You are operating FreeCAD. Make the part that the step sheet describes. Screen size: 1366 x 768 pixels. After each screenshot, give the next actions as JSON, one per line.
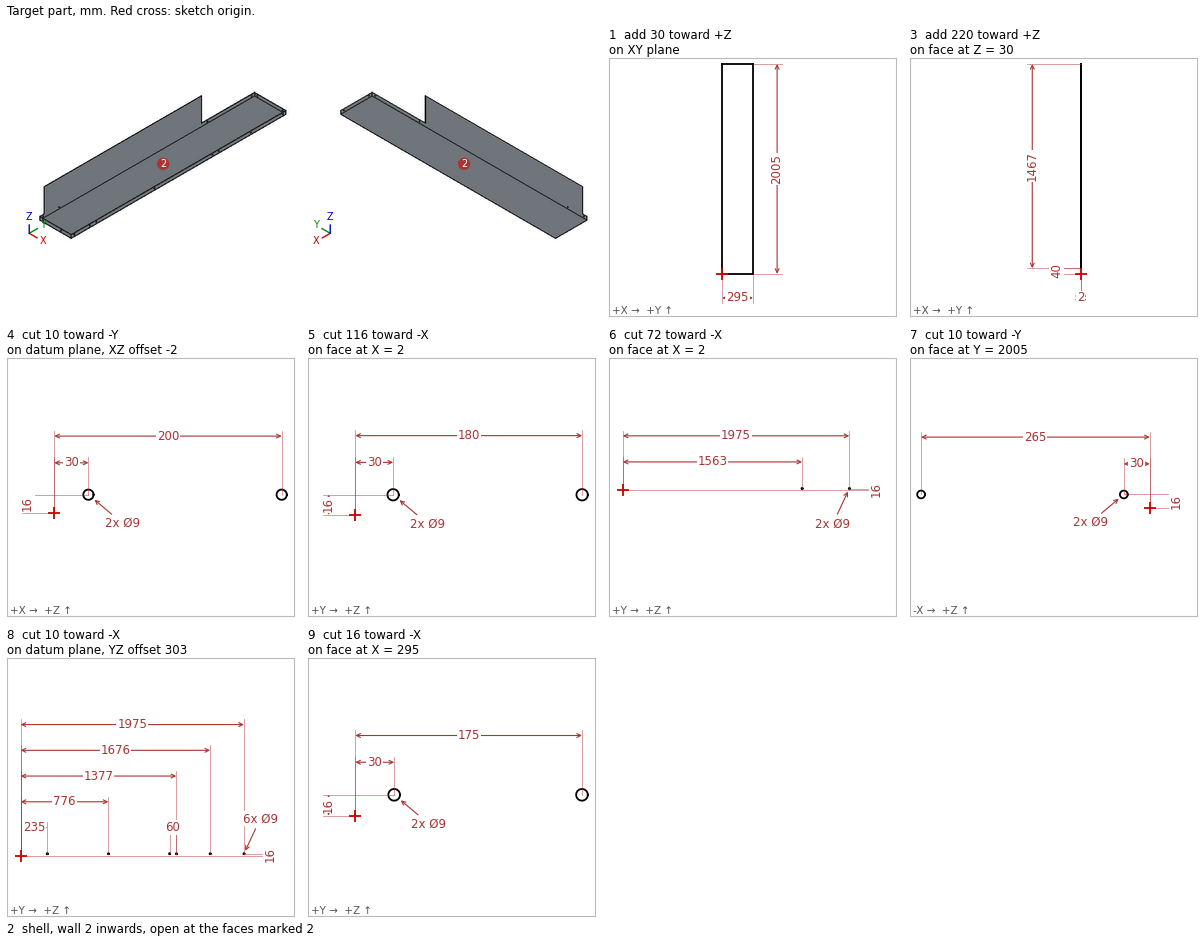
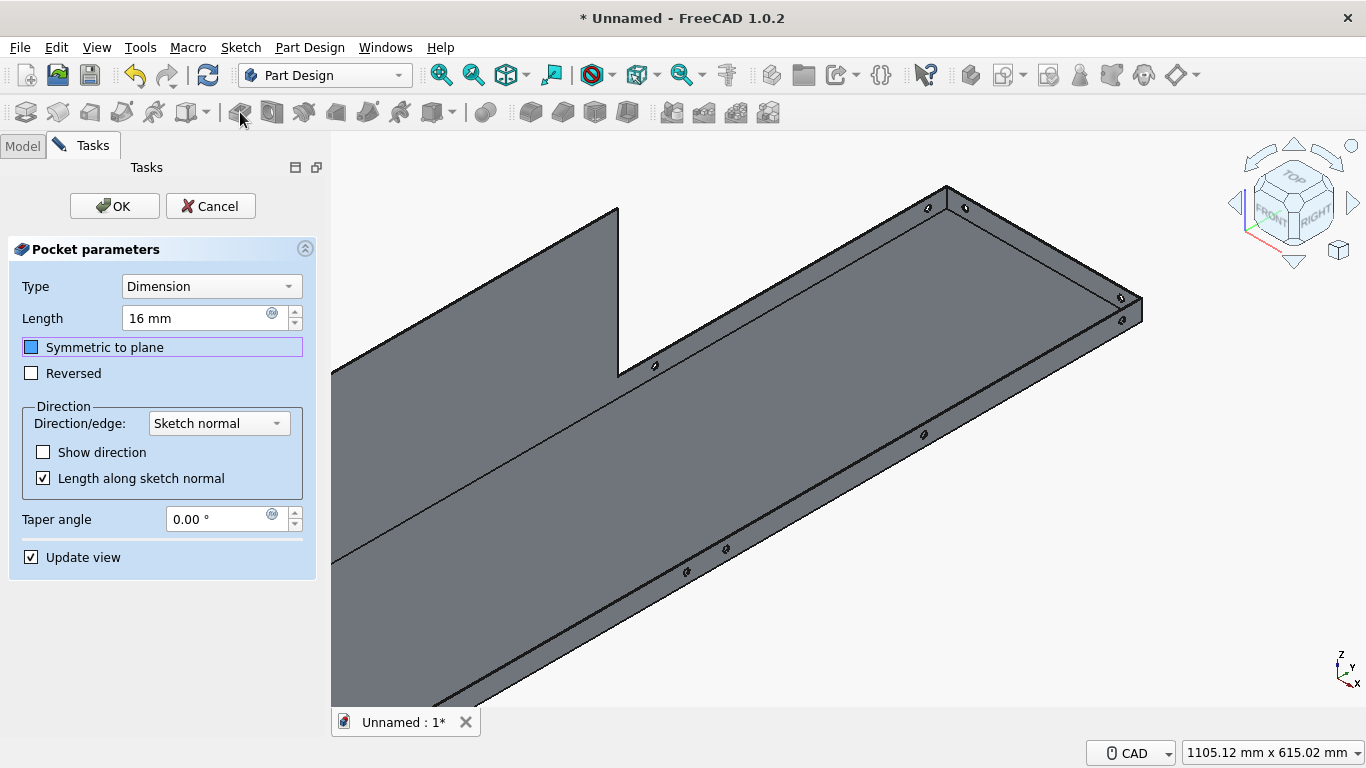
{"action": "left_click", "coordinate": [115, 206]}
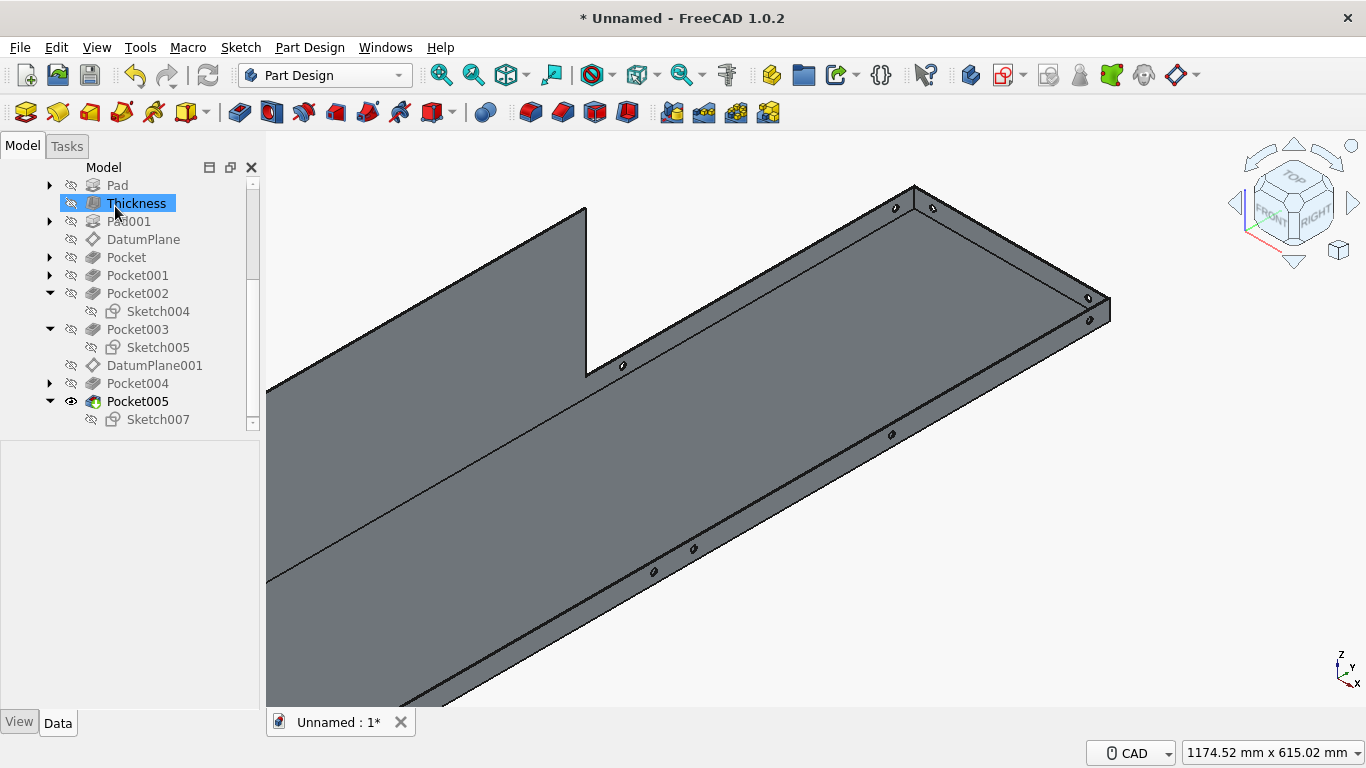
{"action": "left_click", "coordinate": [442, 76]}